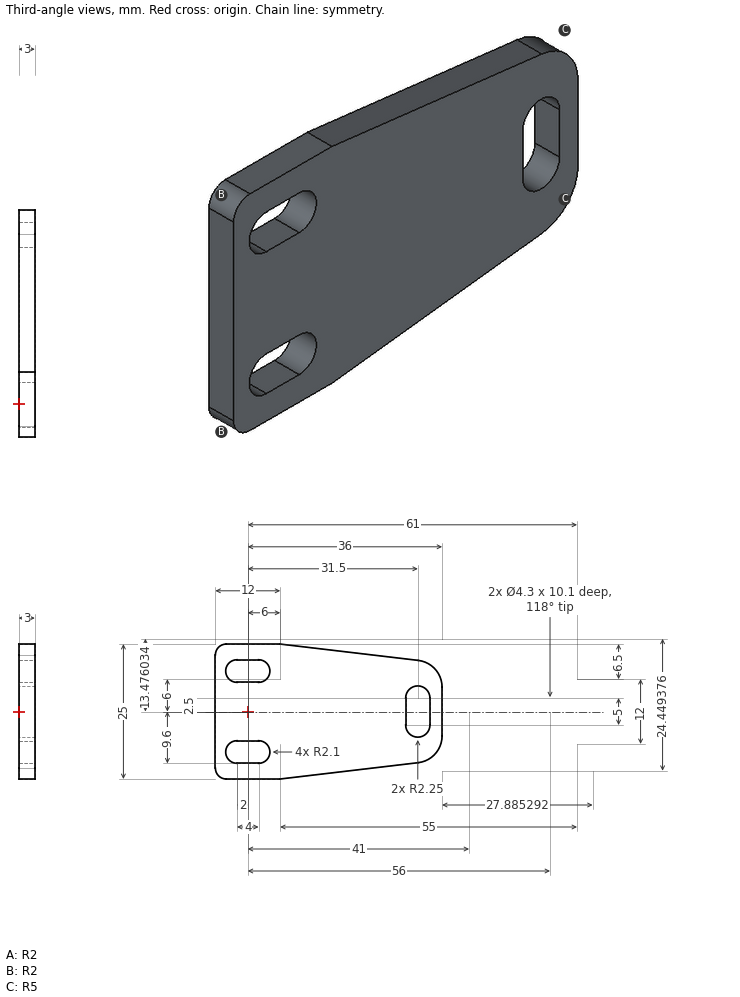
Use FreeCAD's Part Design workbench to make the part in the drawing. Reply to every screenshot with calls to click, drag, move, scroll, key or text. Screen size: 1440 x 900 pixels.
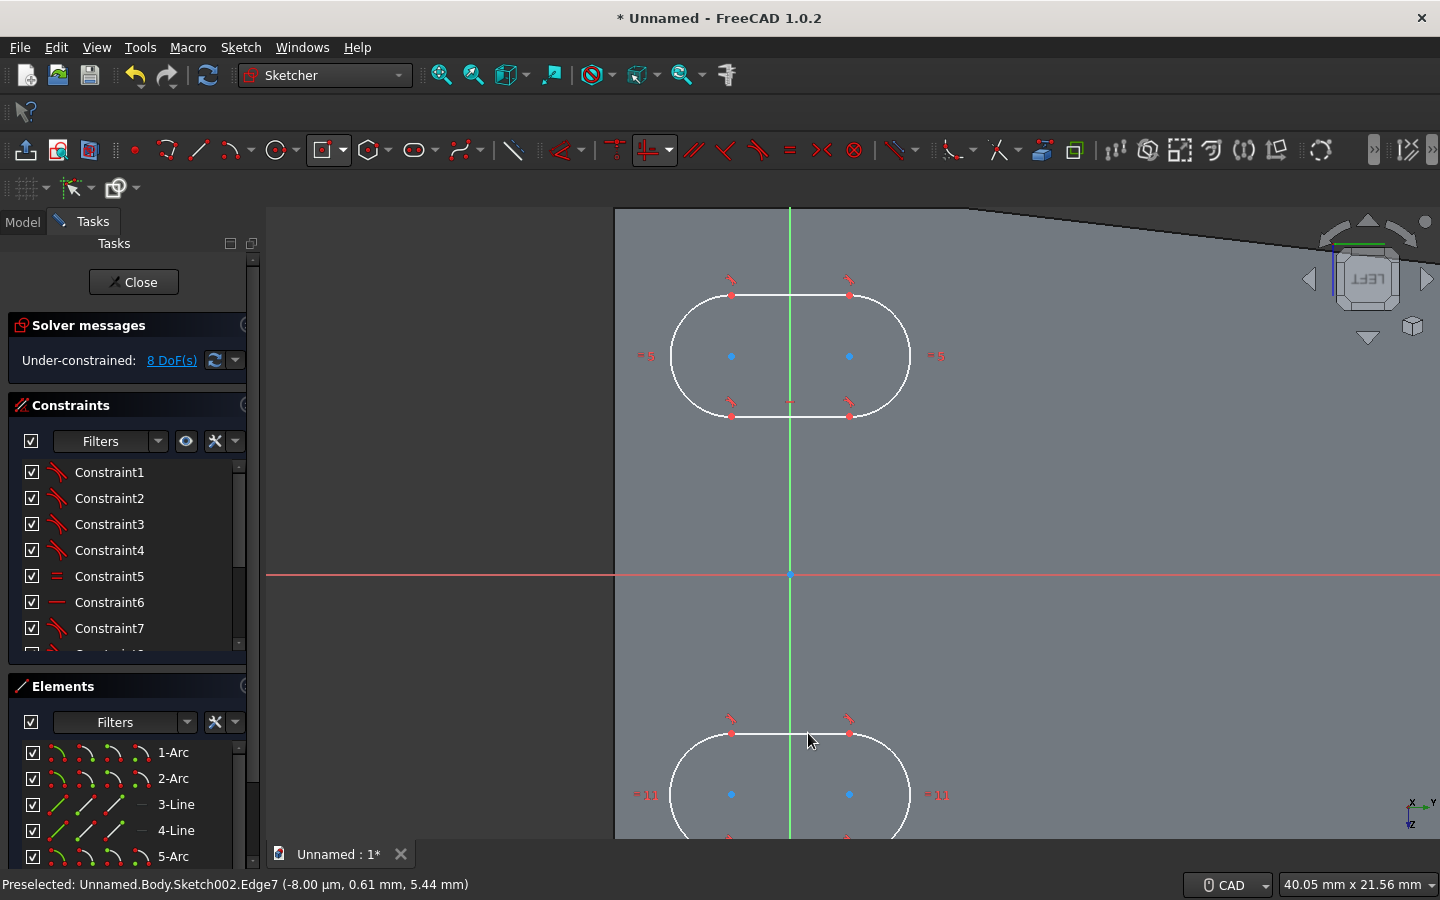
click(682, 320)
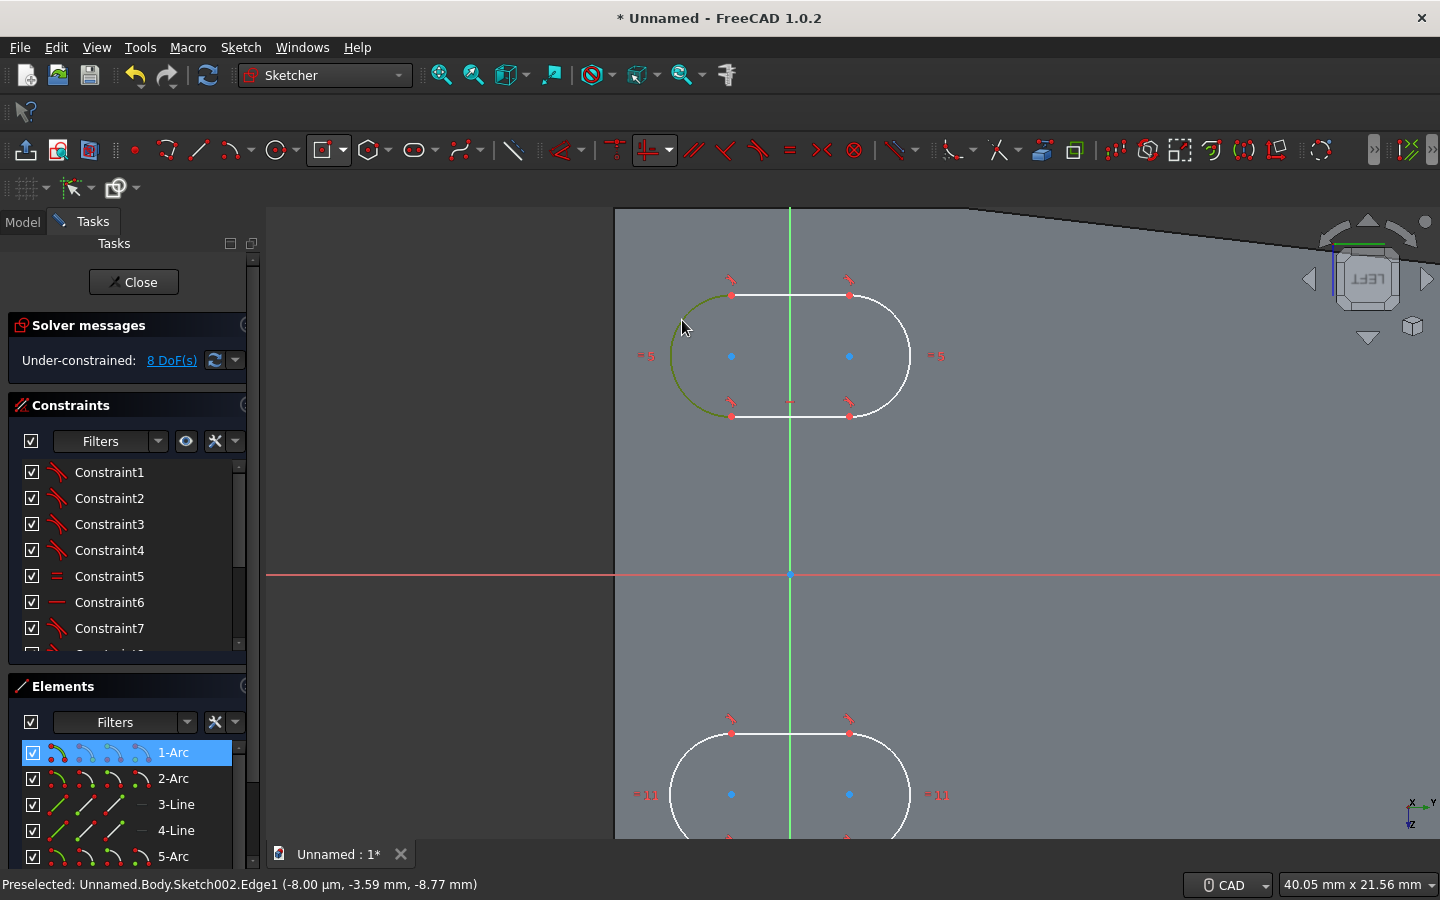
click(682, 759)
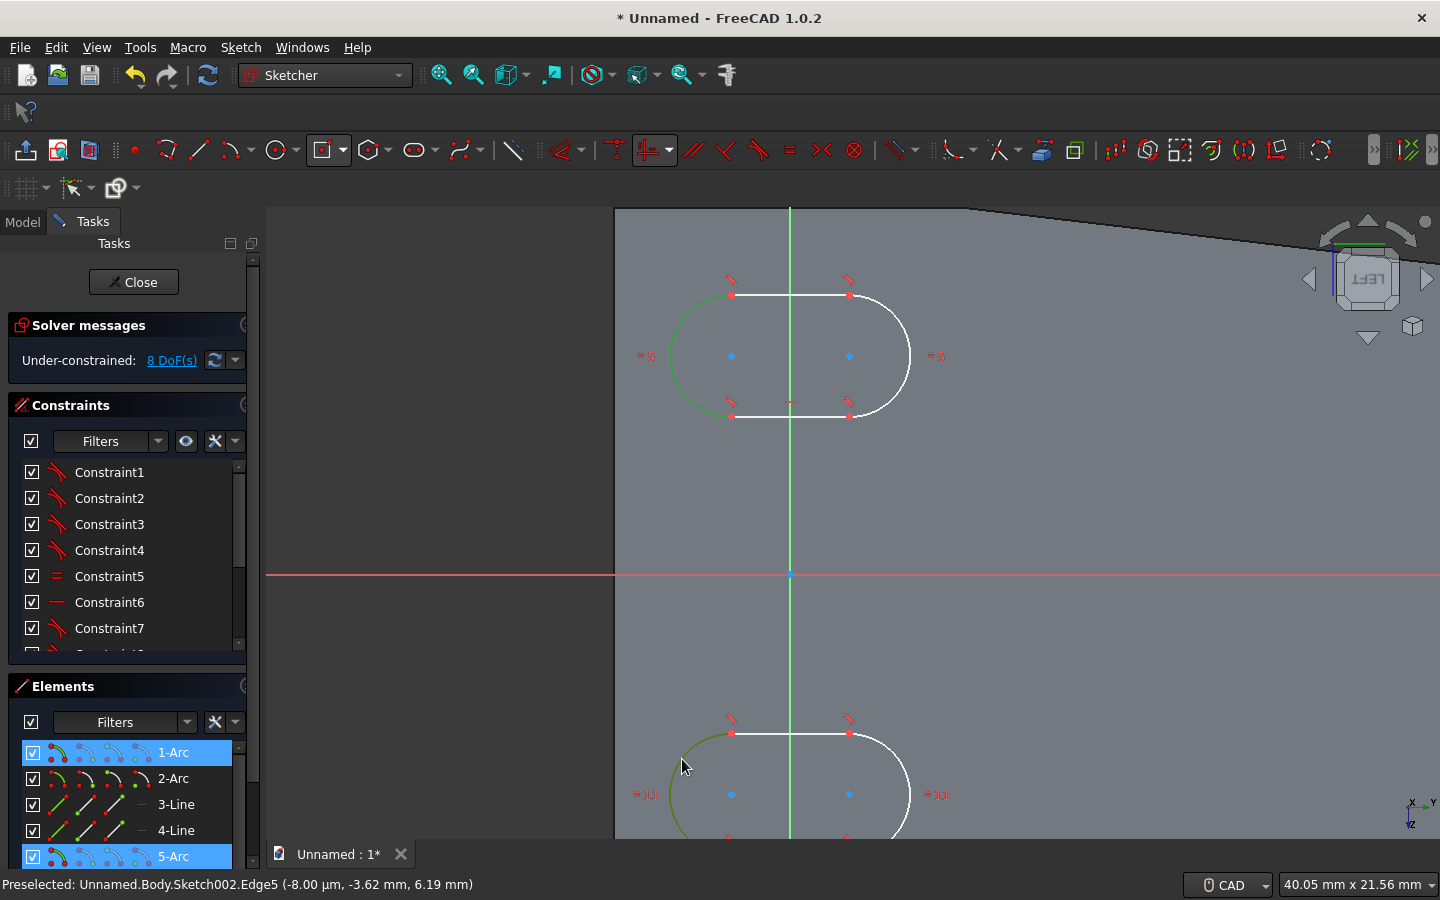
key(e)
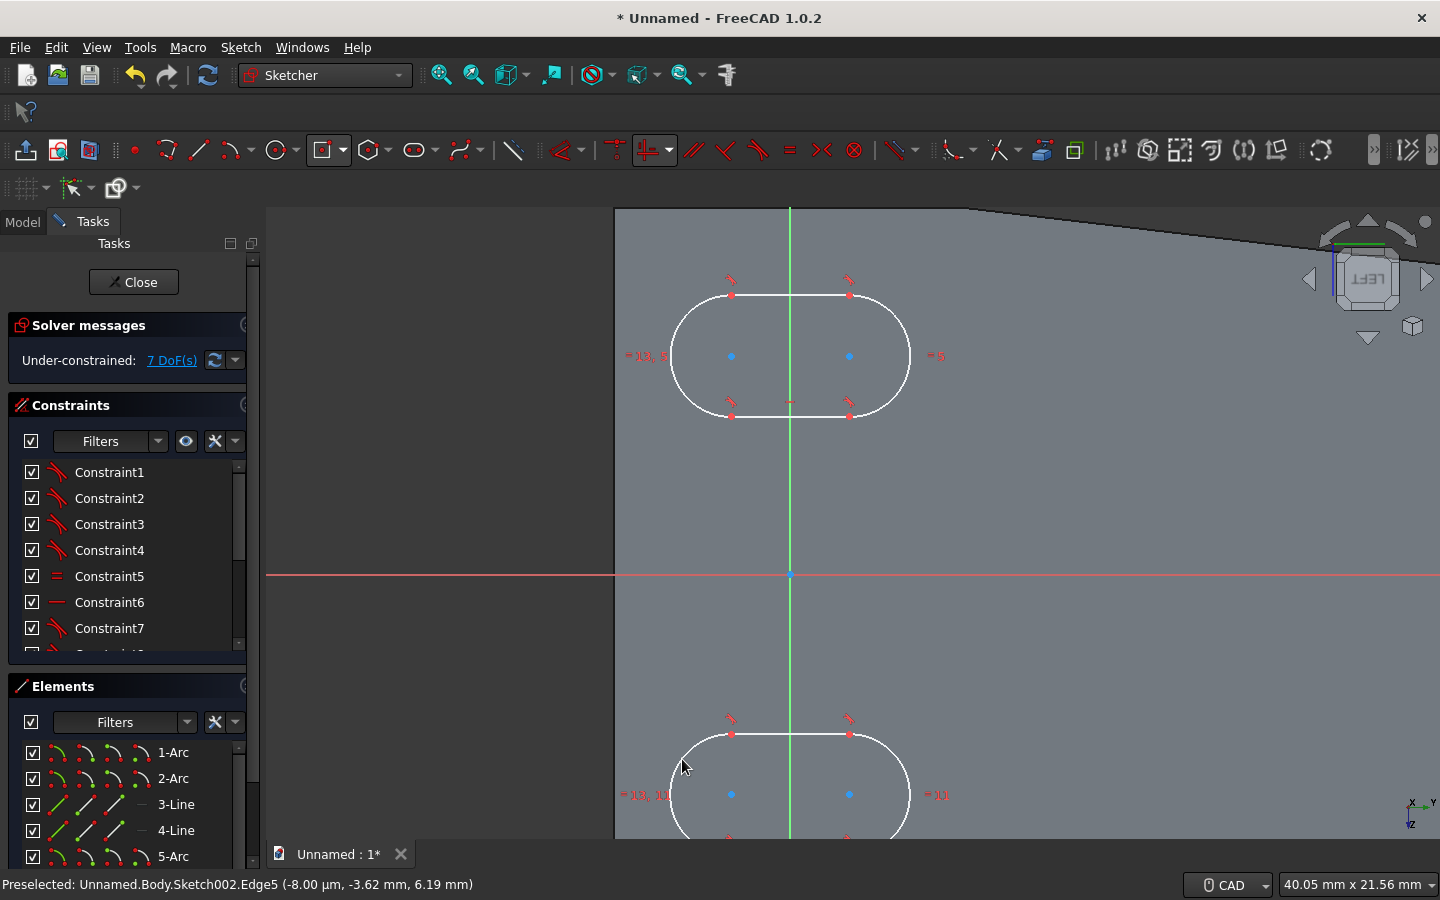
click(732, 356)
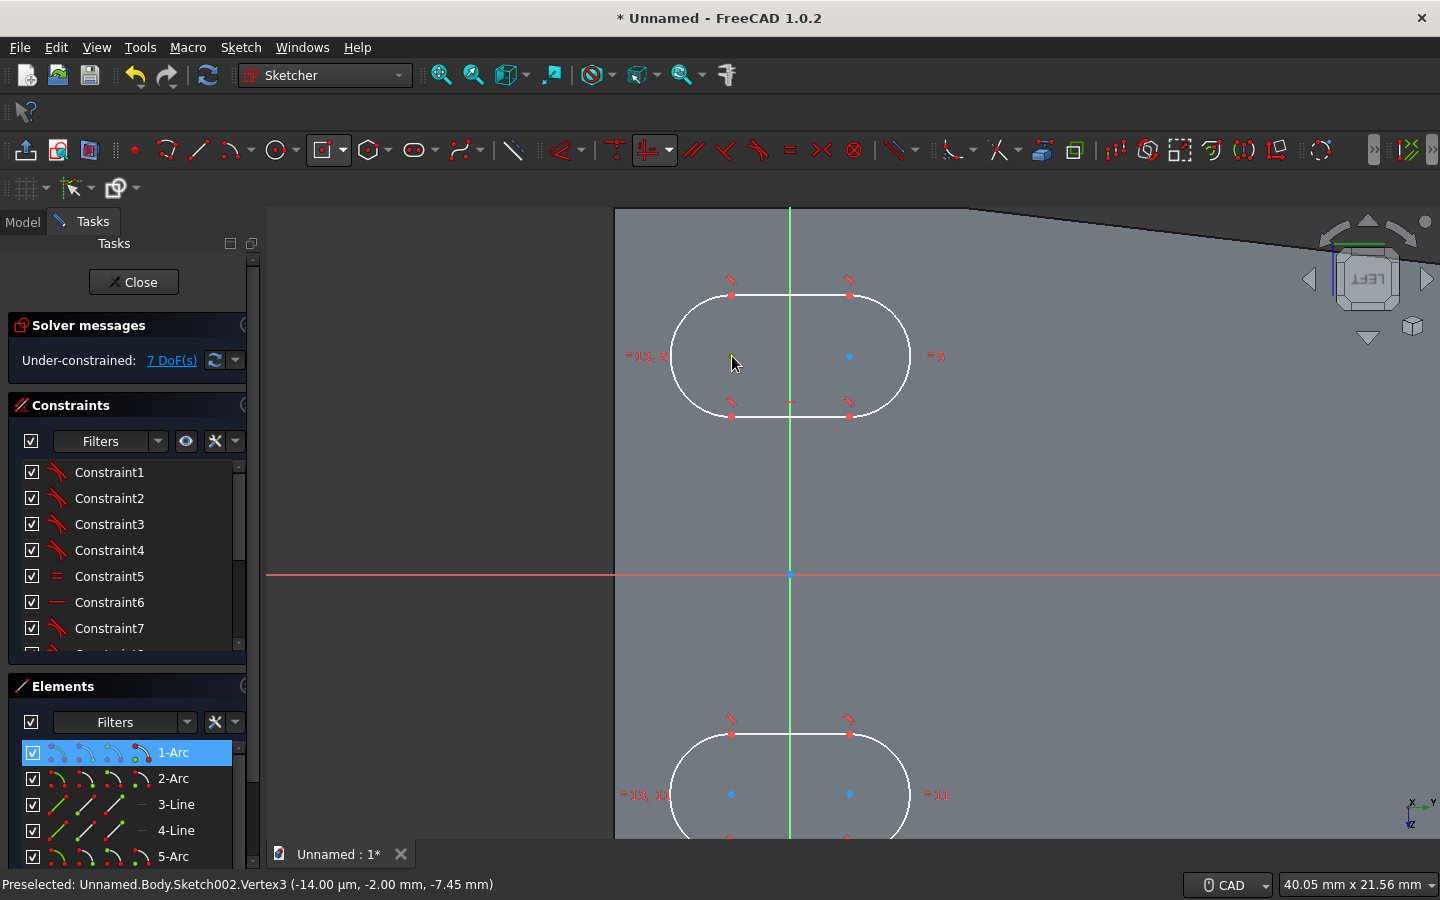
click(731, 795)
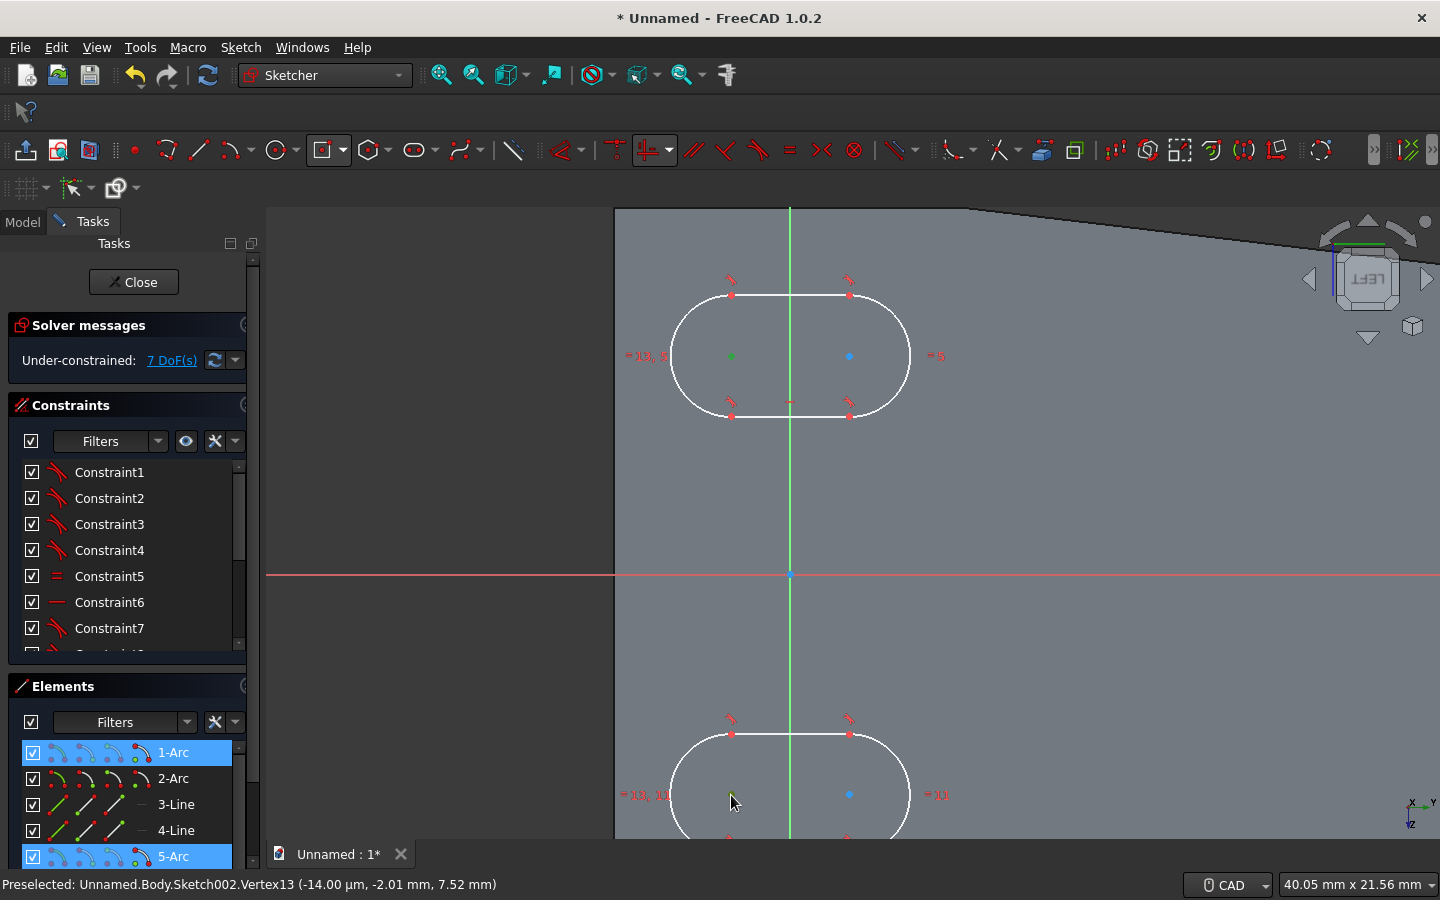
click(364, 575)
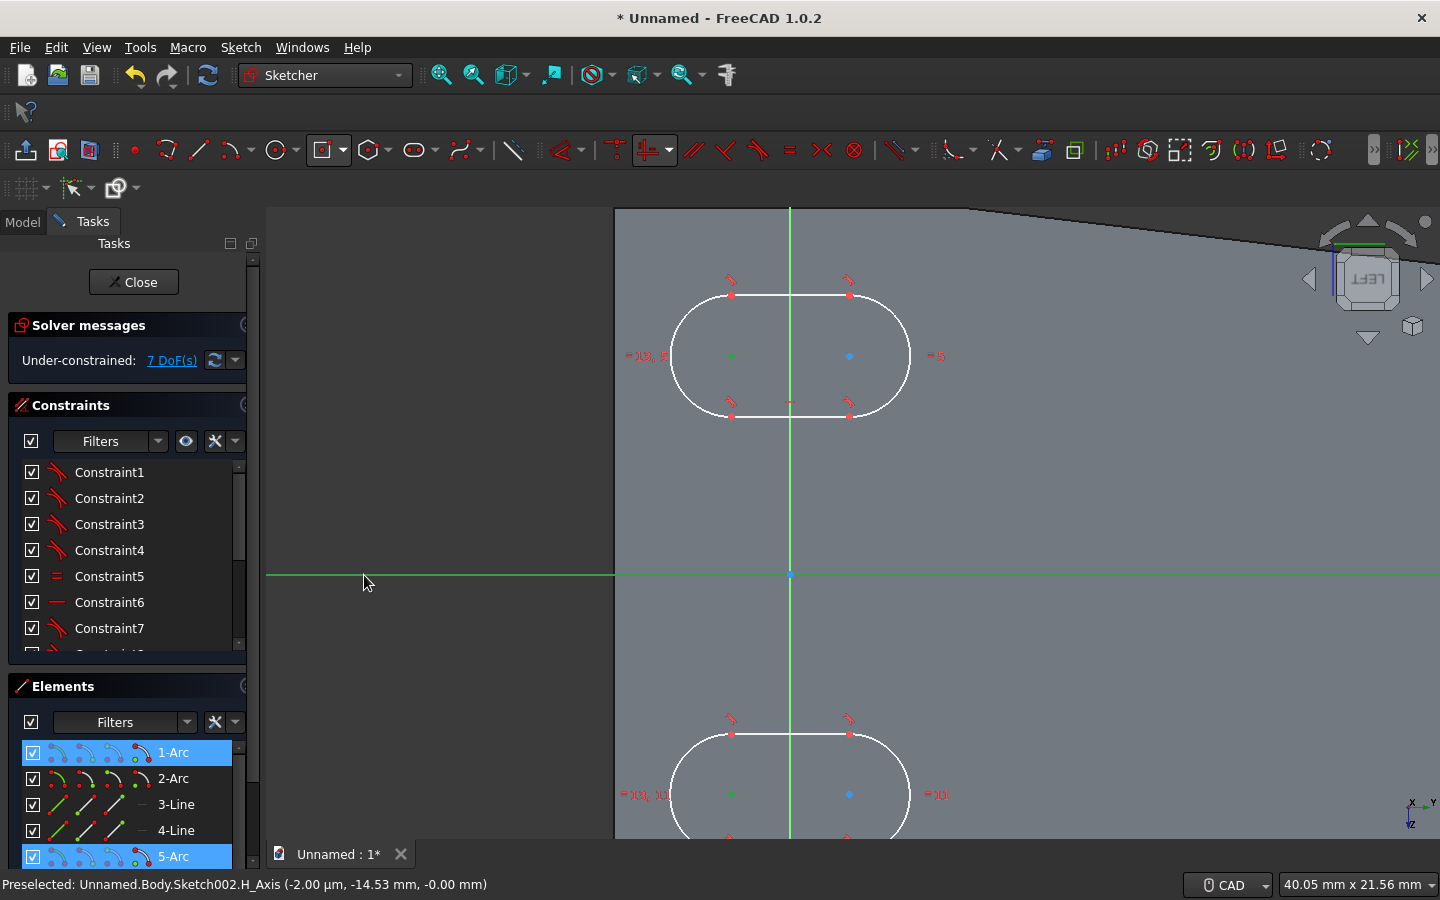
key(s)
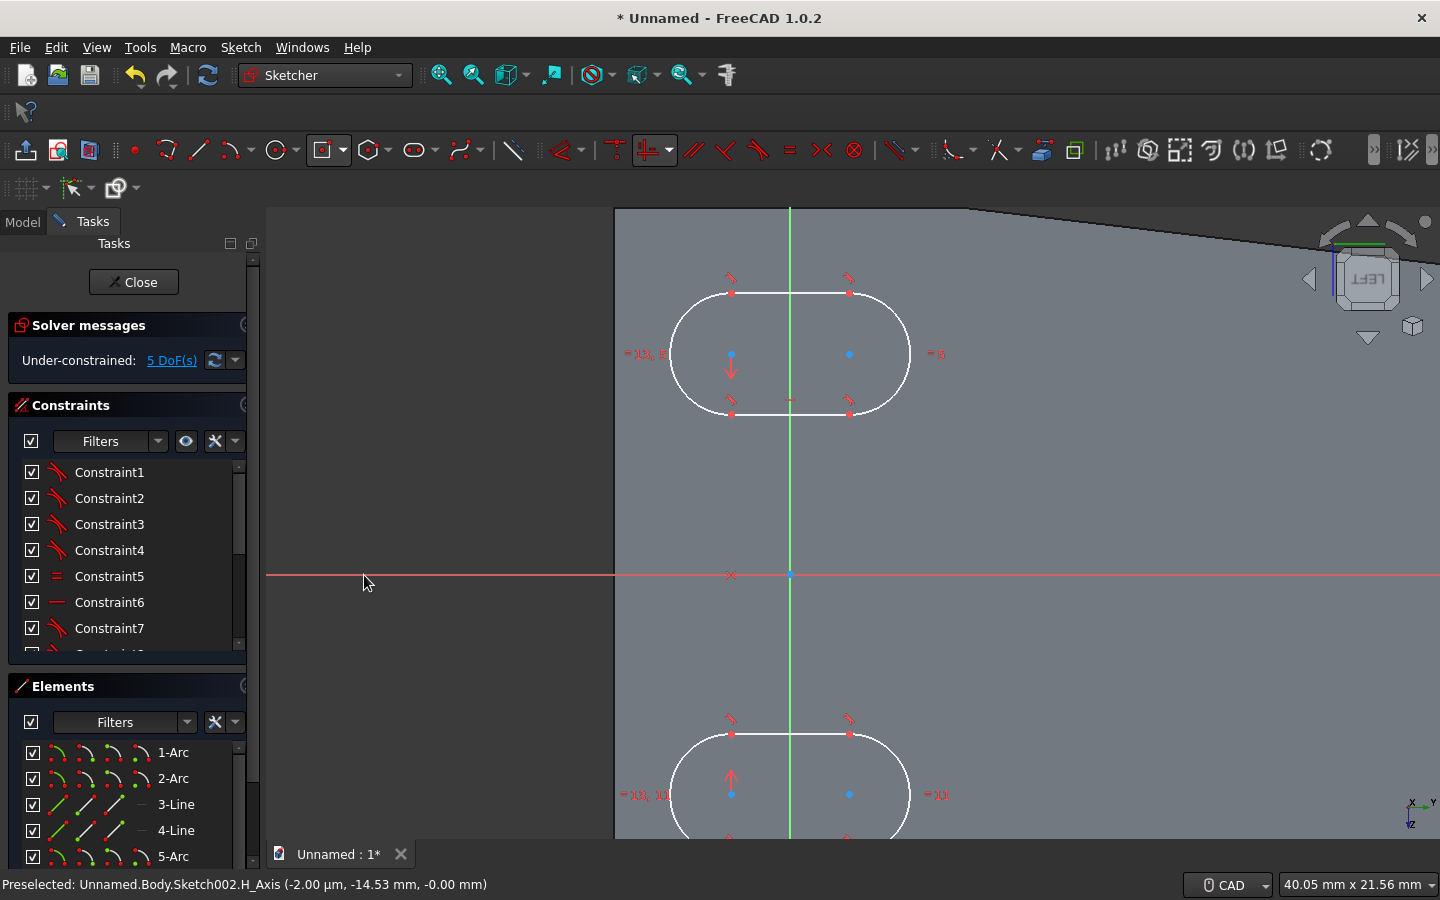
key(d)